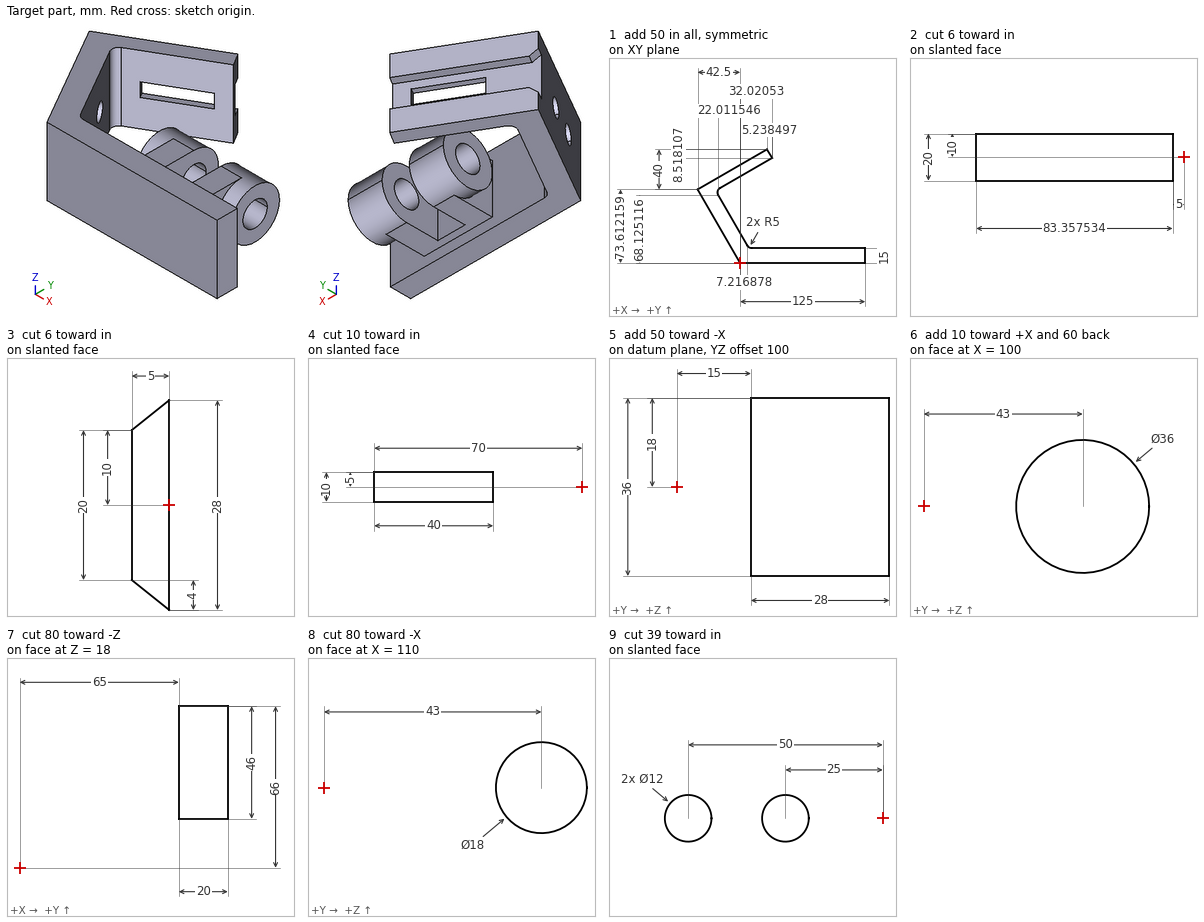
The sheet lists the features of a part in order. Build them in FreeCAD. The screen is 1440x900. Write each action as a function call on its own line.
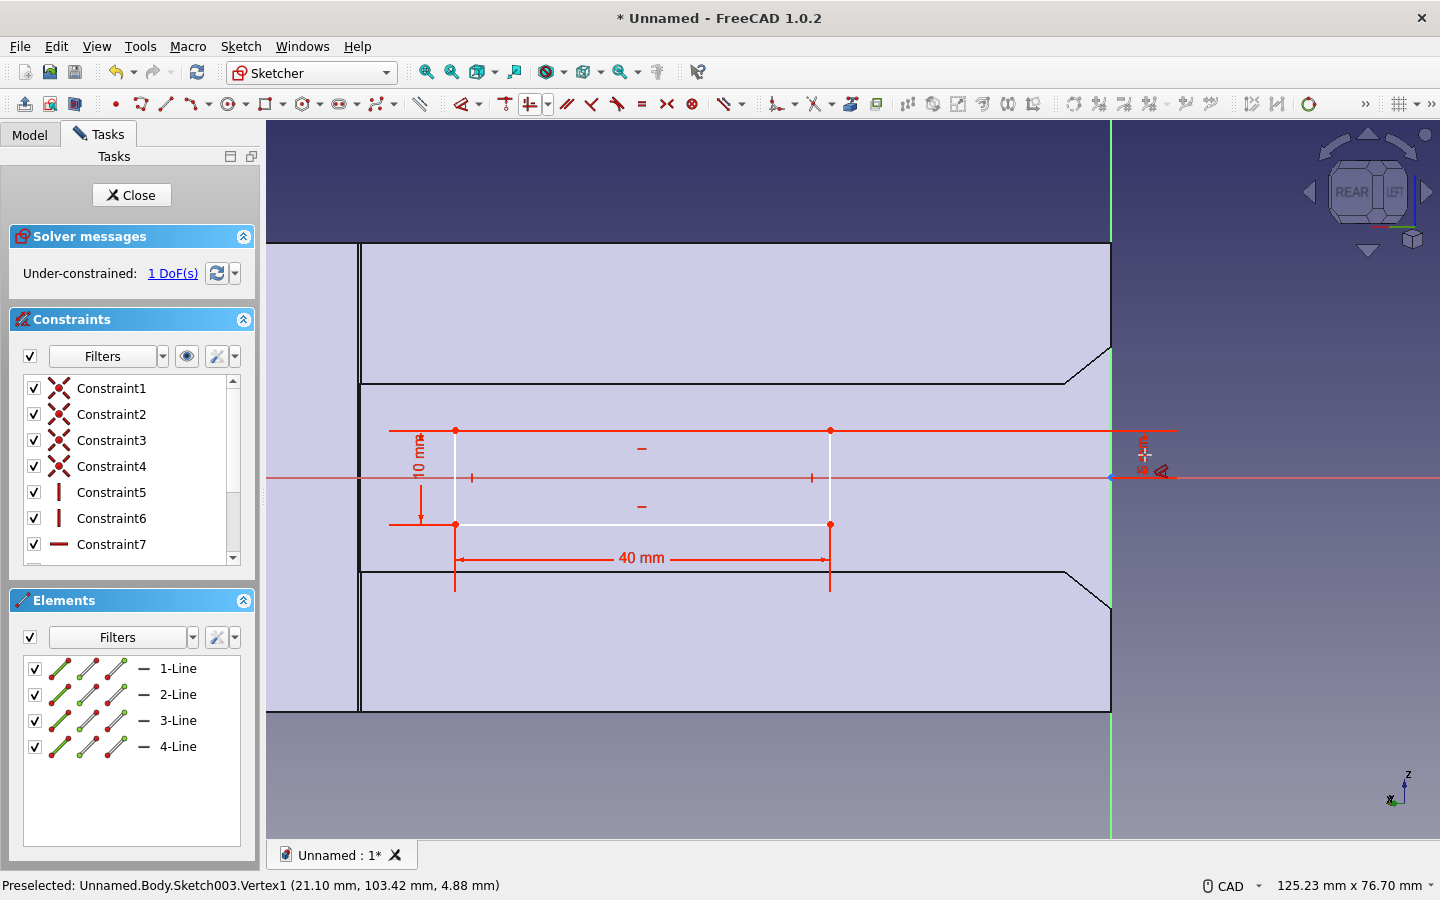
click(455, 431)
click(783, 397)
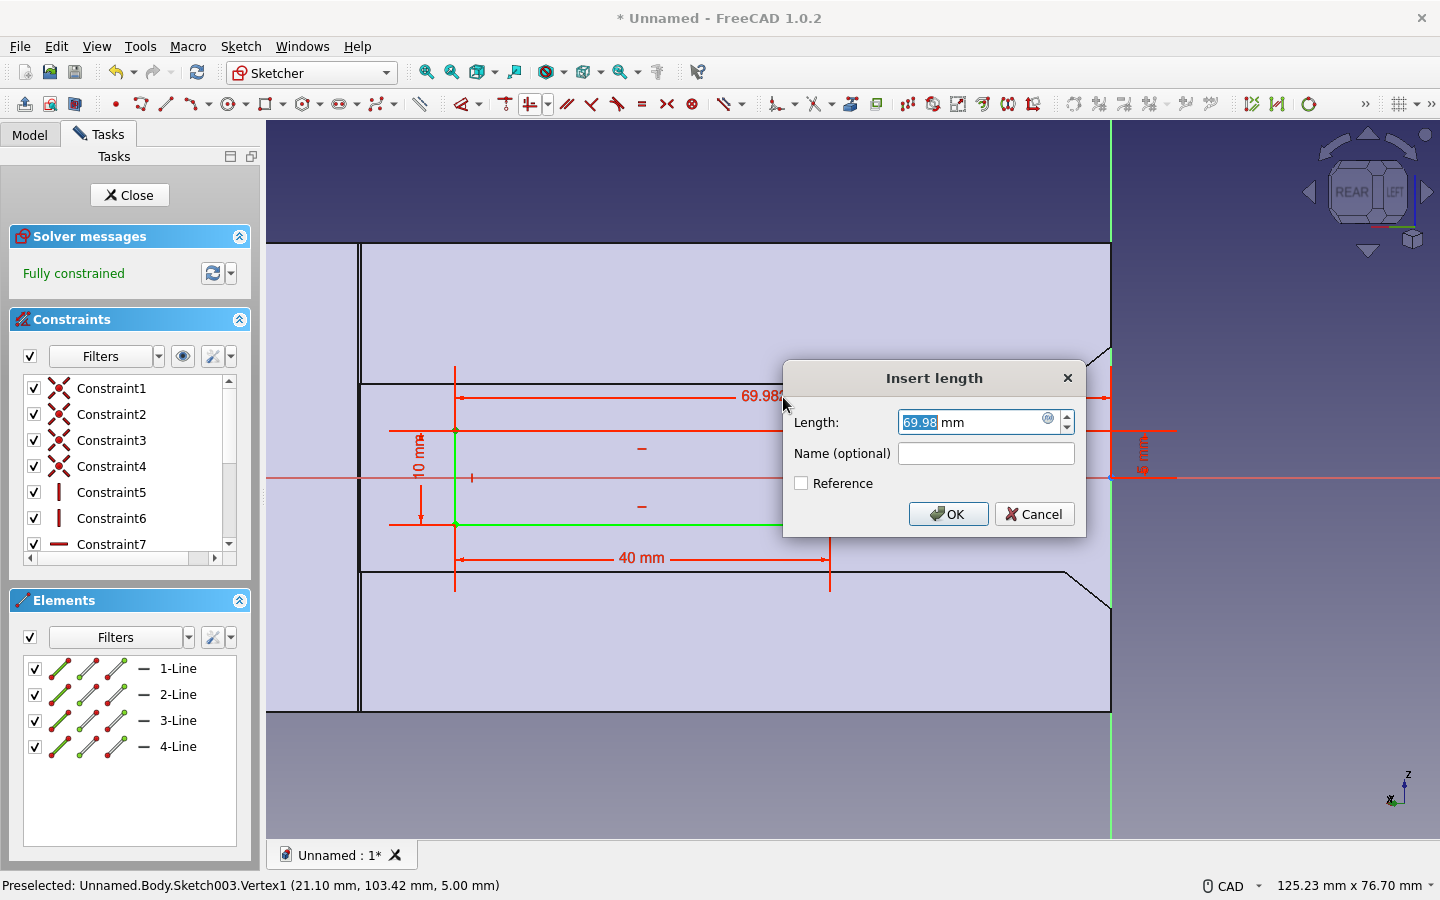
text(70)
key(Return)
key(Escape)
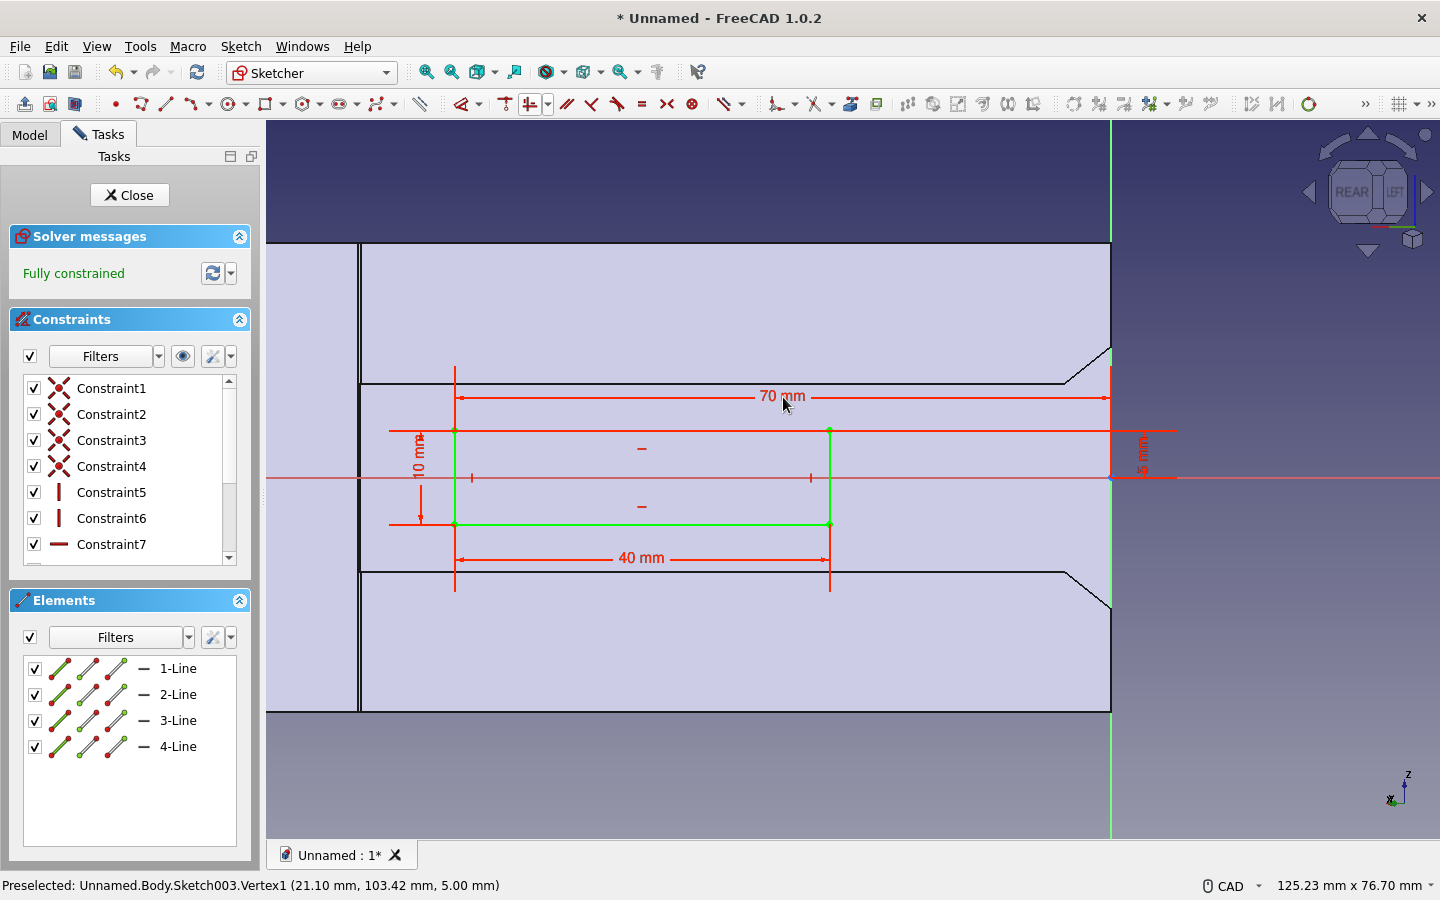
click(130, 195)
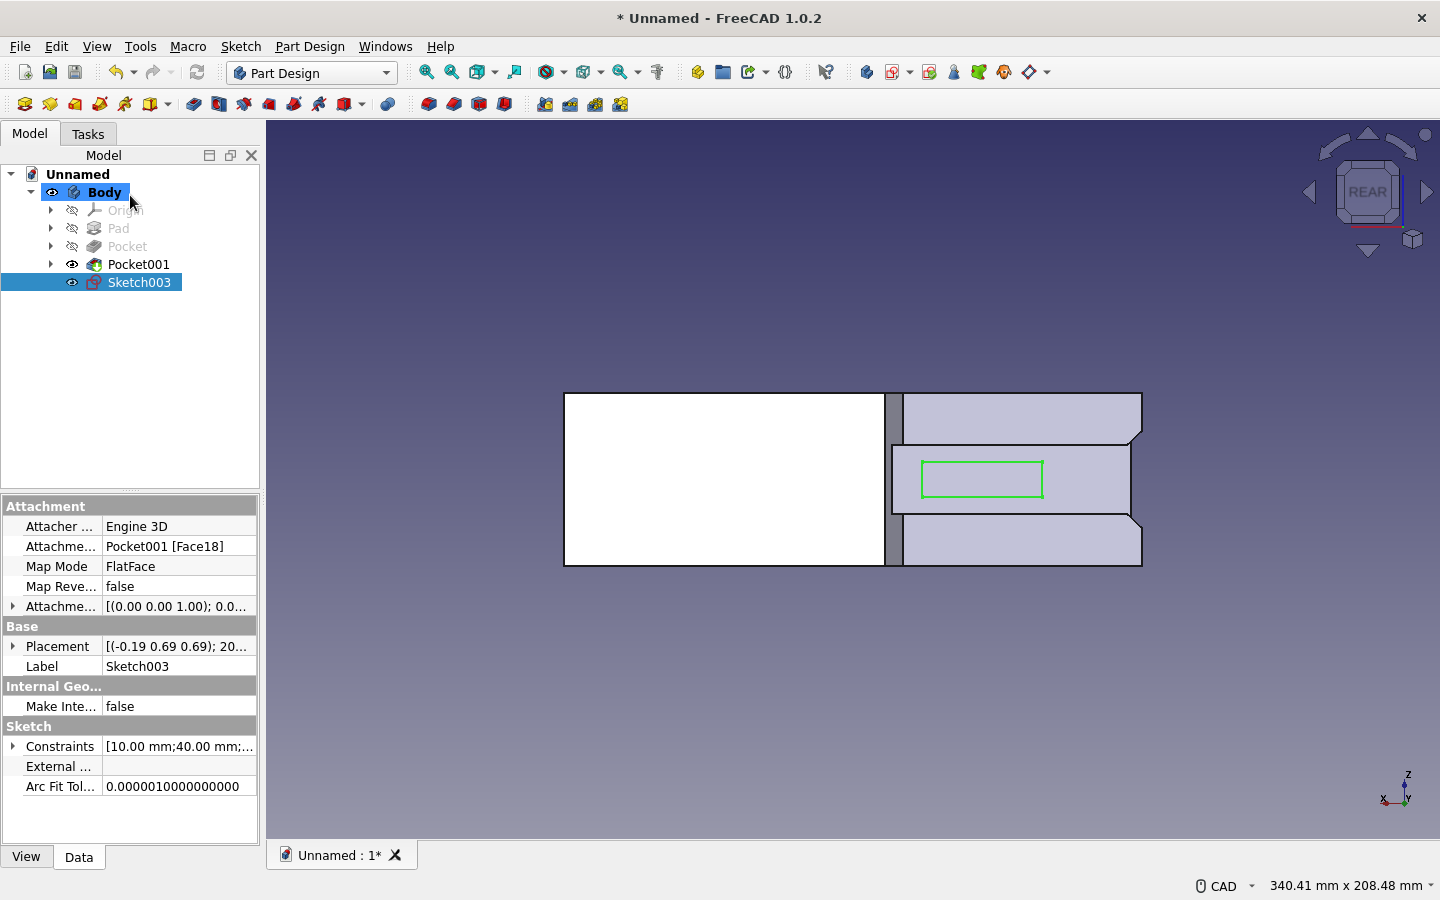
click(194, 104)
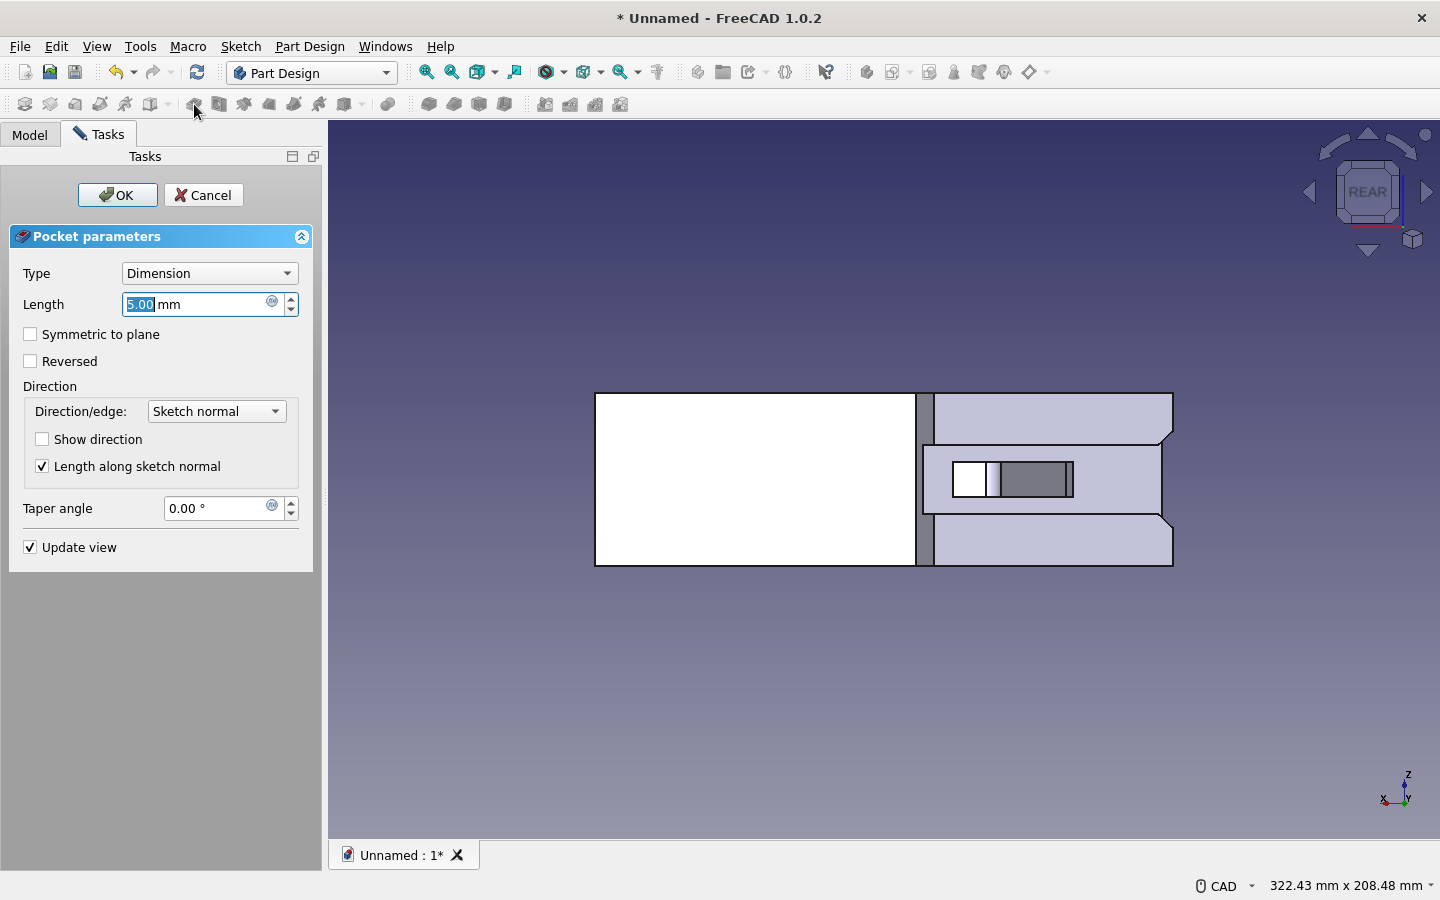
text(10)
key(Tab)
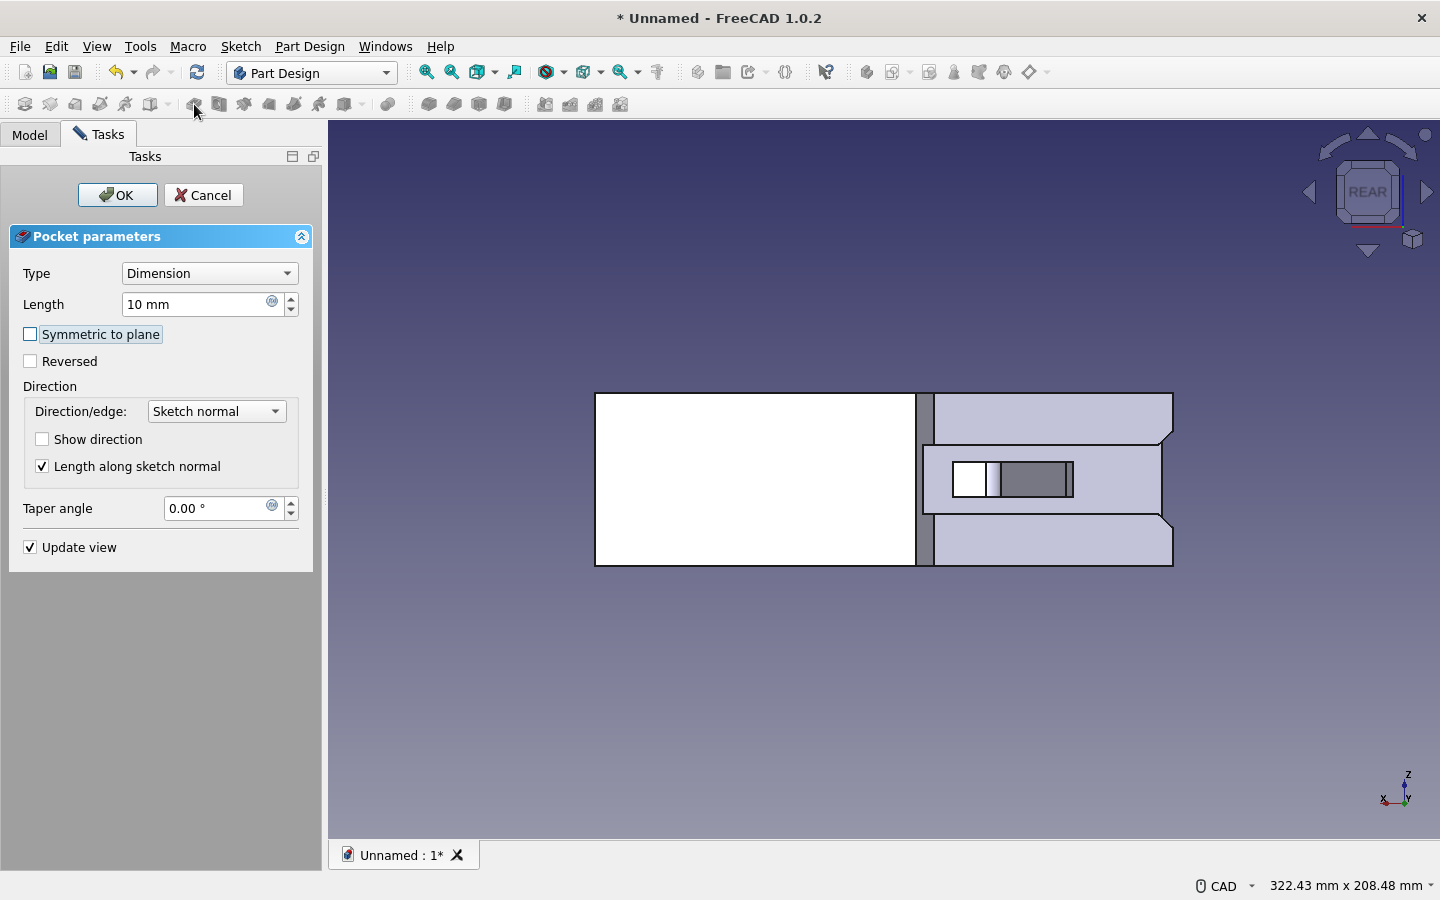
click(118, 195)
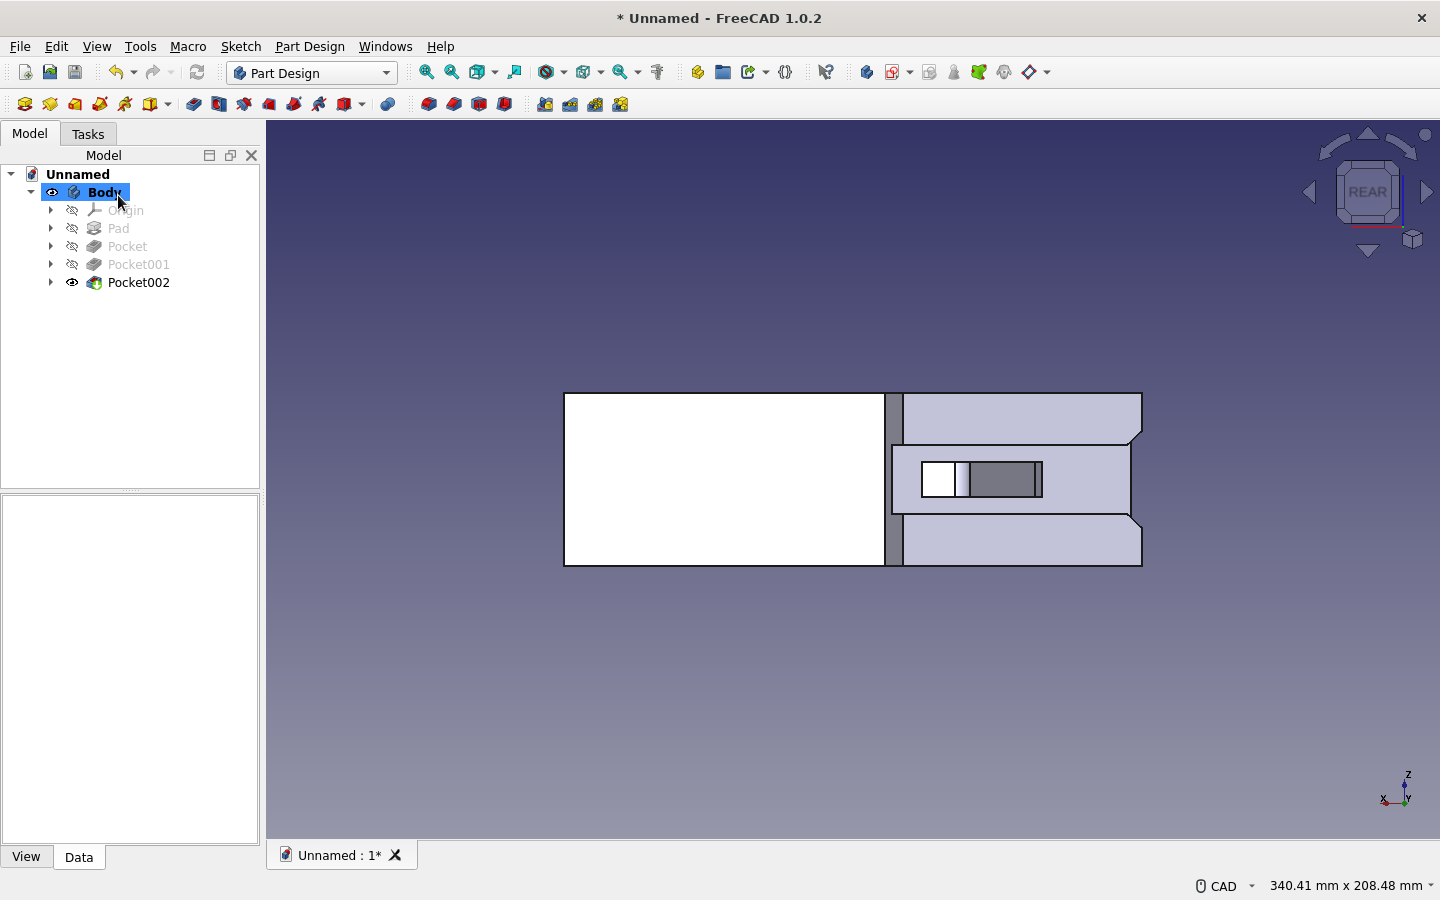
click(51, 210)